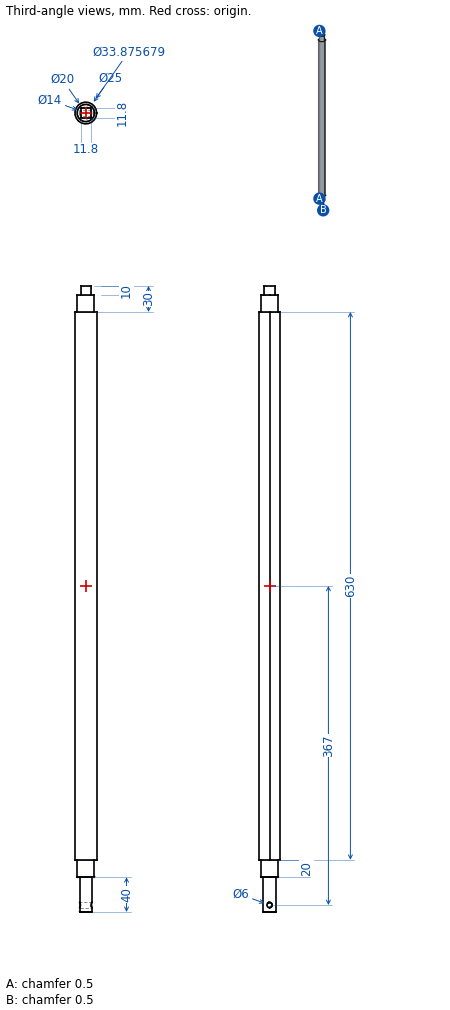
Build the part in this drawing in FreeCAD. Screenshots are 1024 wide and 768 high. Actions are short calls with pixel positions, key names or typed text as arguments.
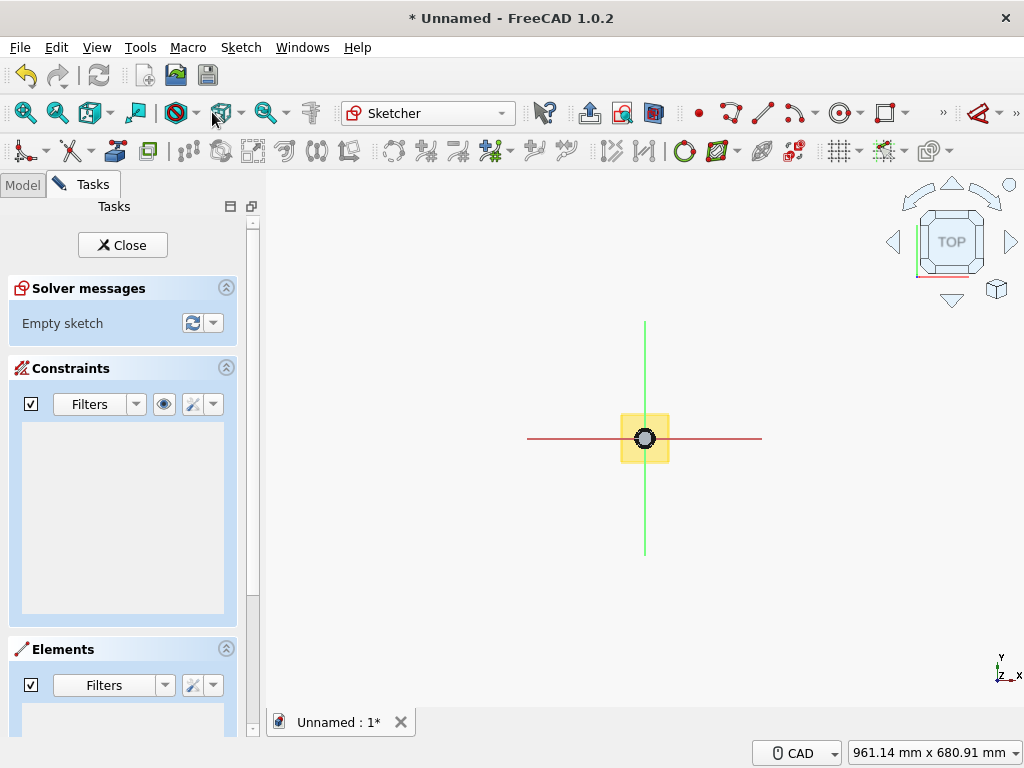
click(654, 114)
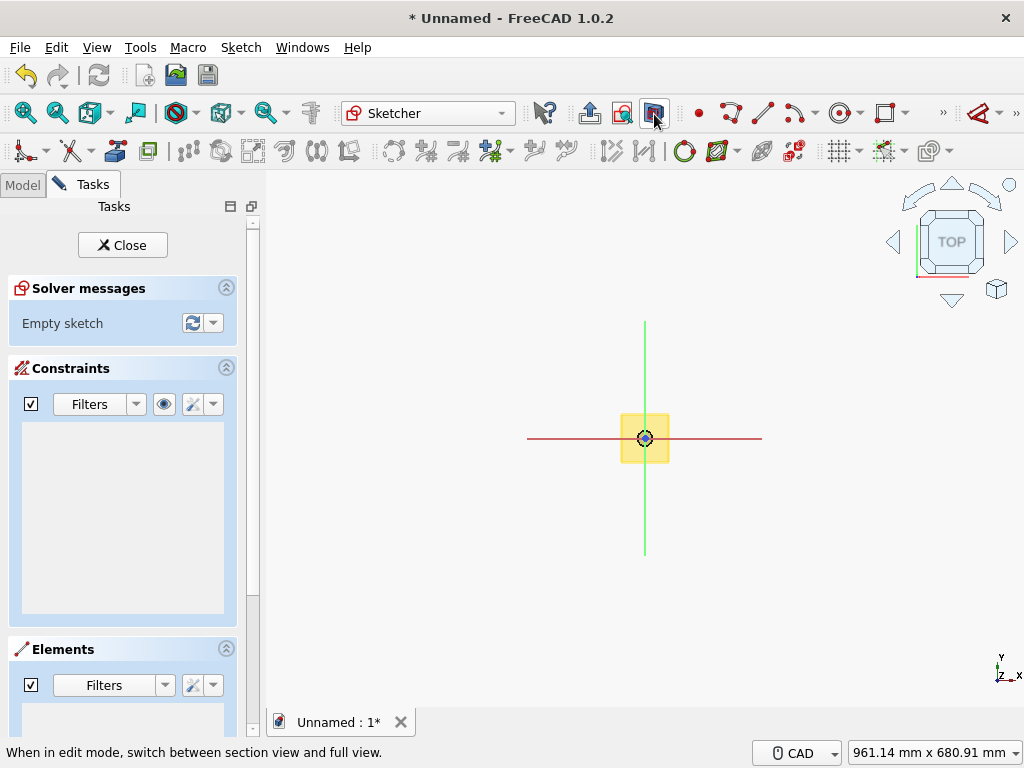
scroll(649, 438, up, 15)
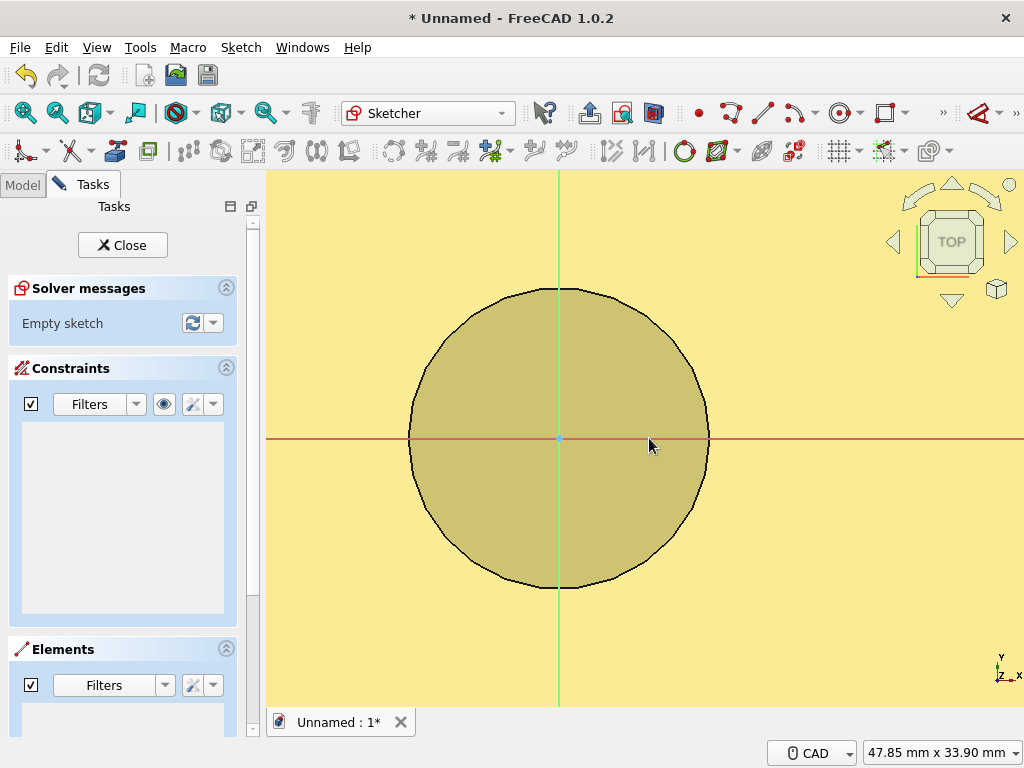
scroll(523, 439, up, 2)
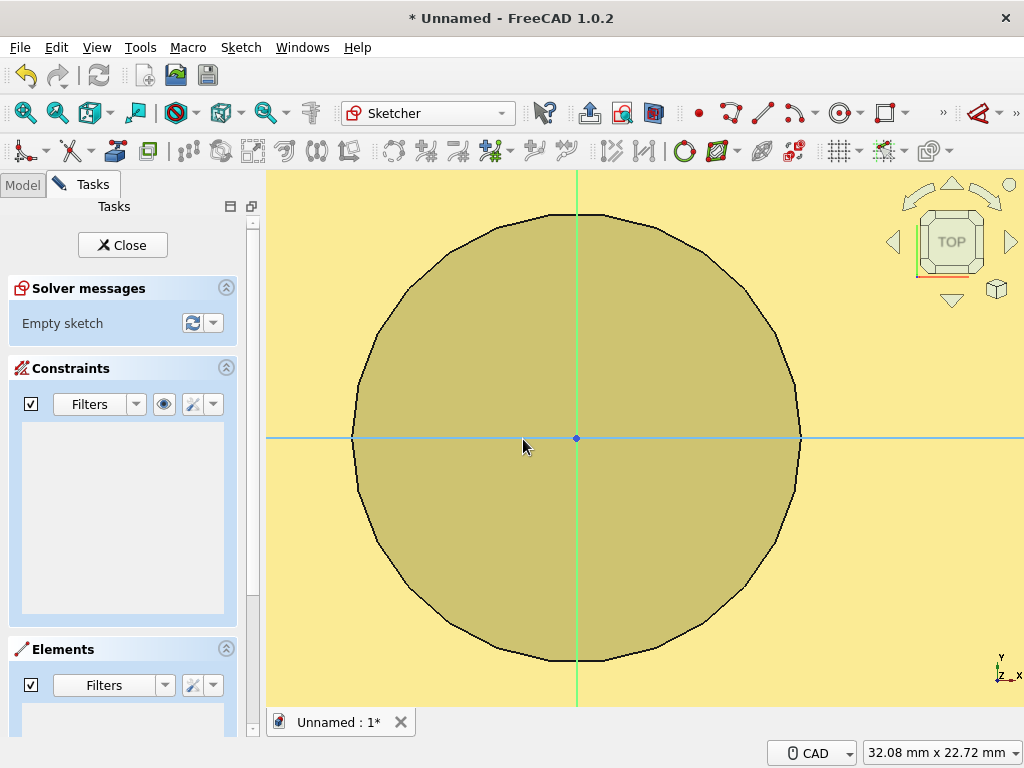
click(840, 114)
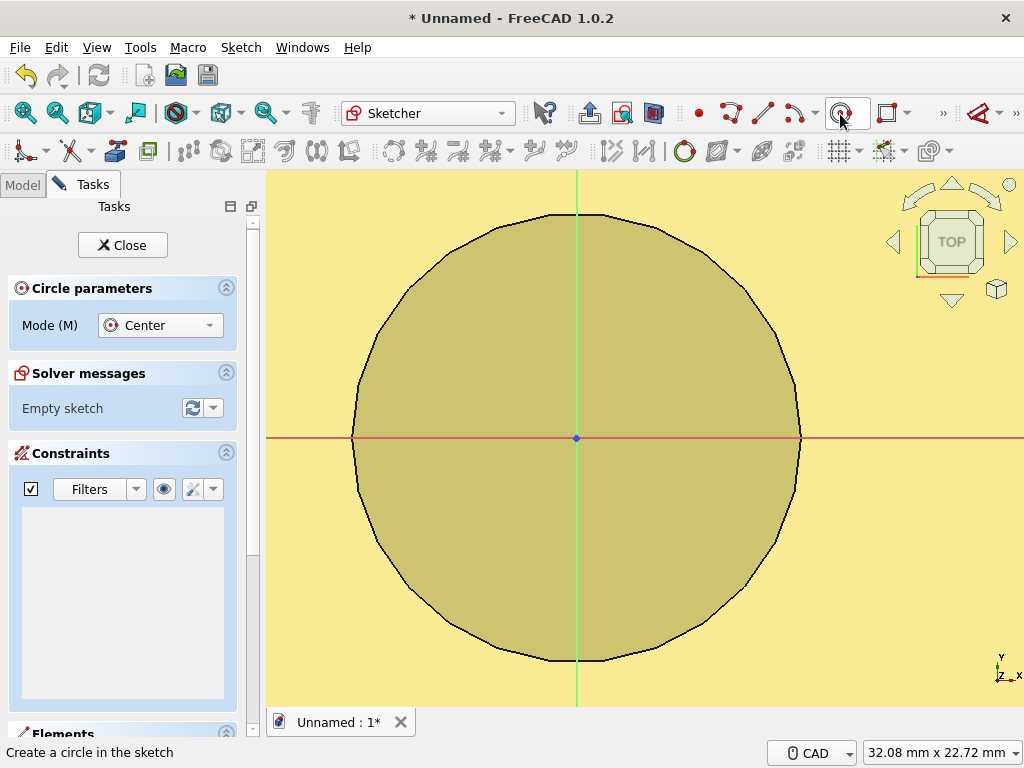
click(577, 438)
move(694, 321)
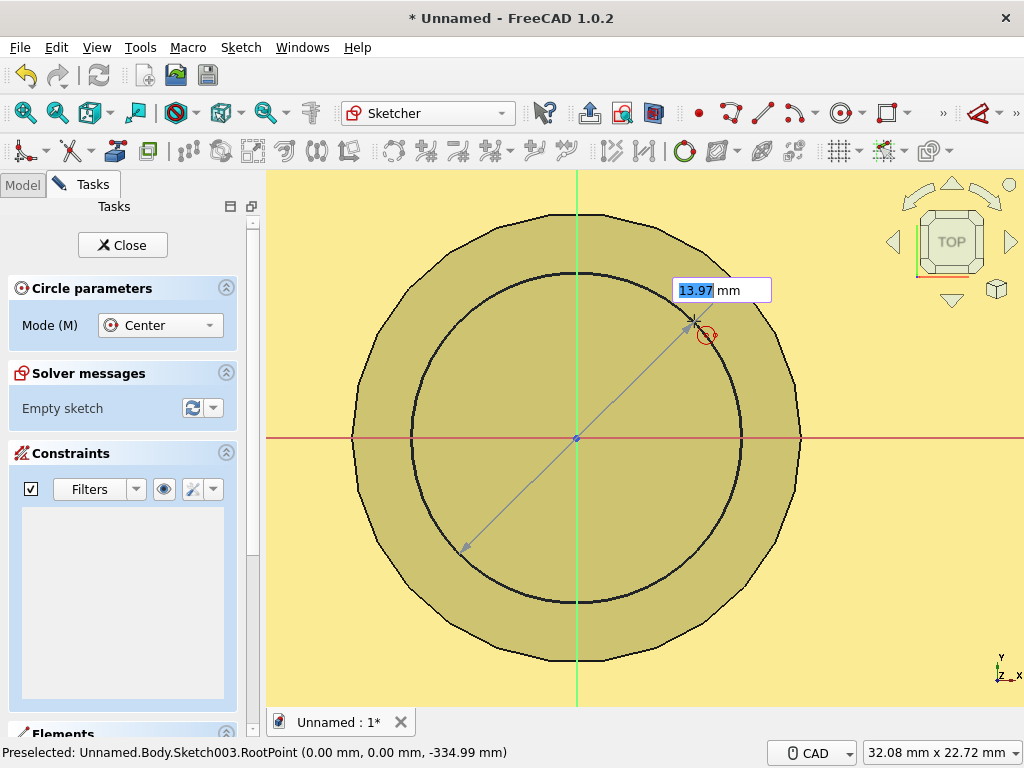
text(14)
key(Return)
key(Escape)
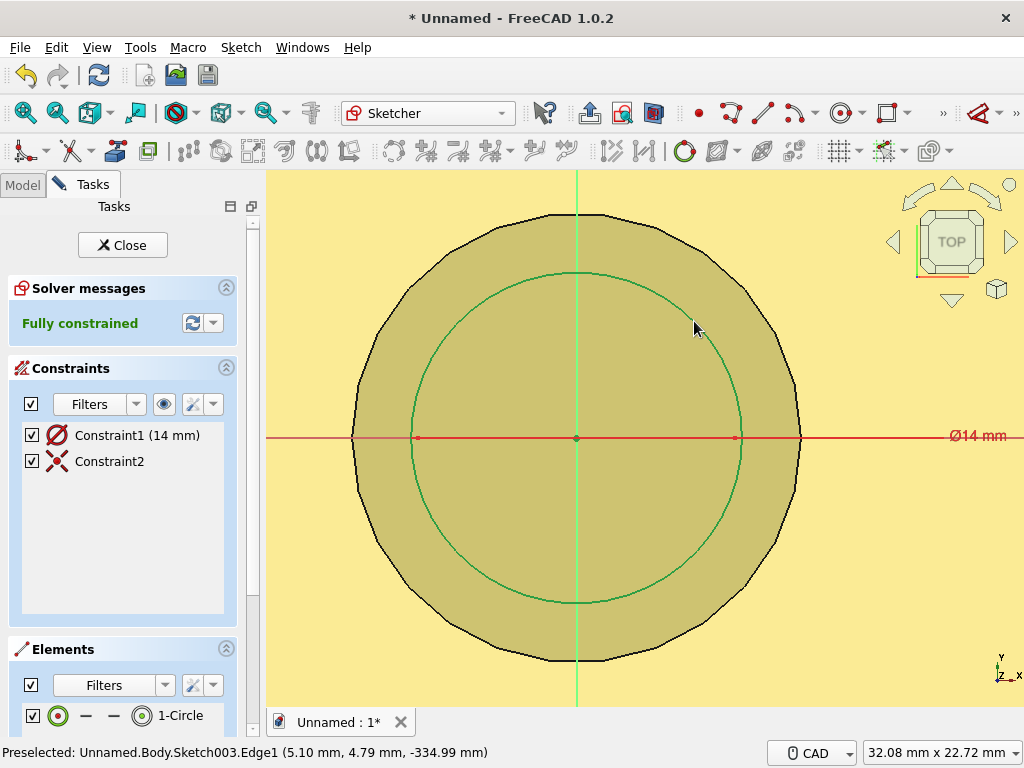
click(123, 245)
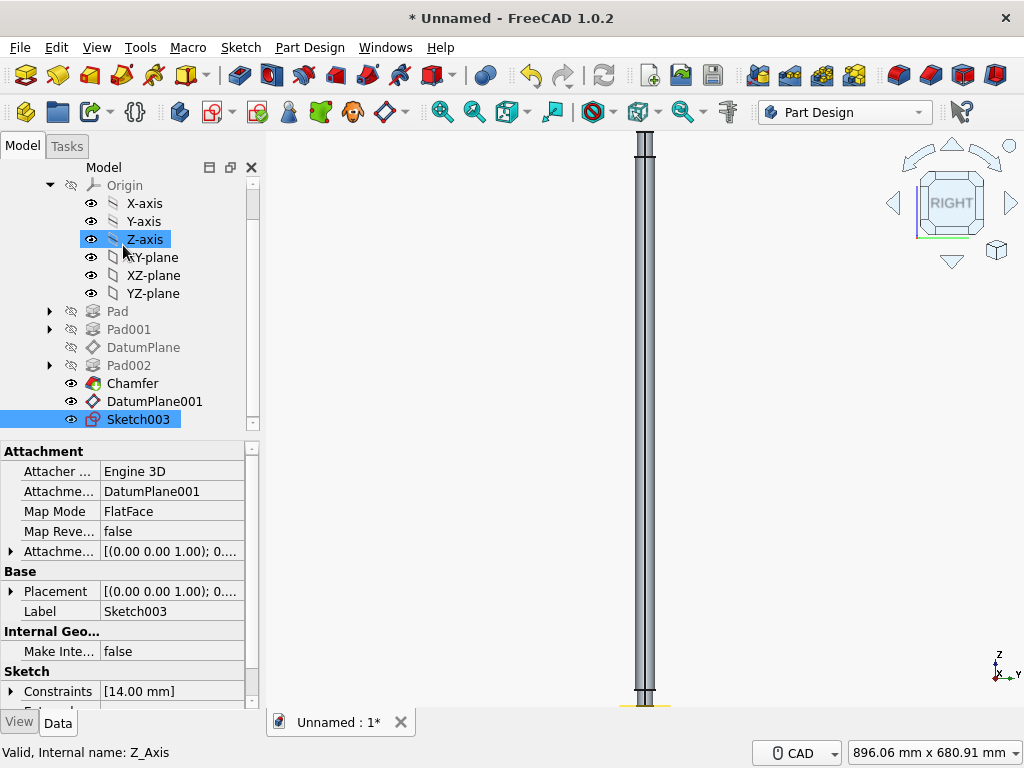
click(26, 76)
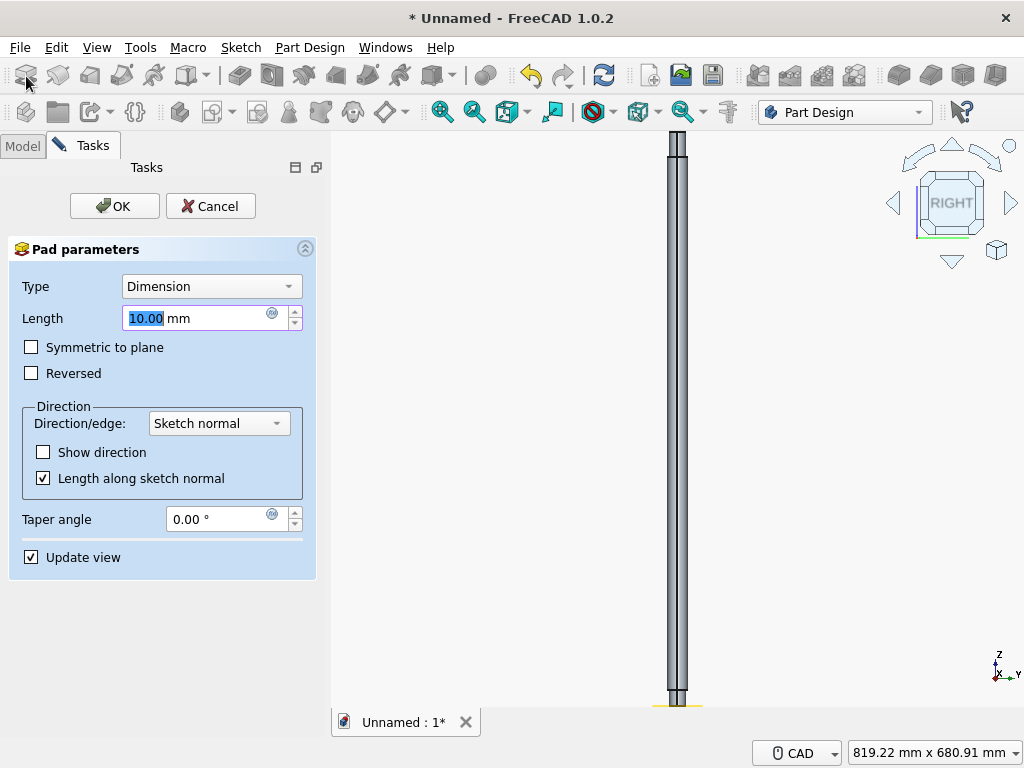
text(40)
key(Tab)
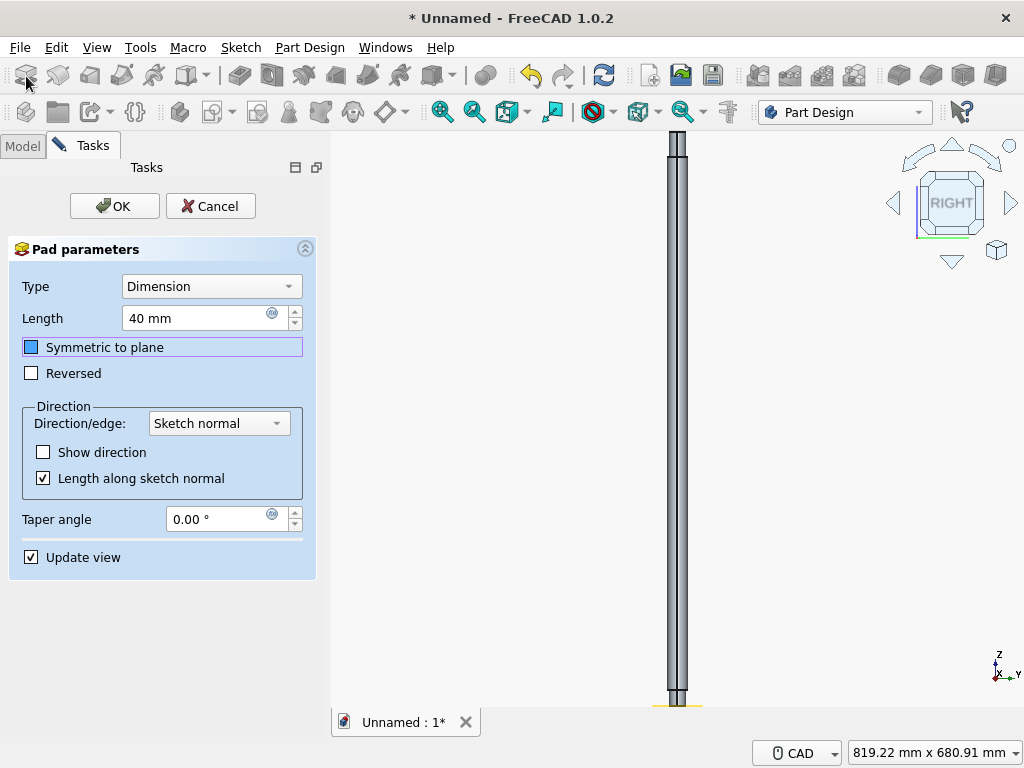
click(30, 373)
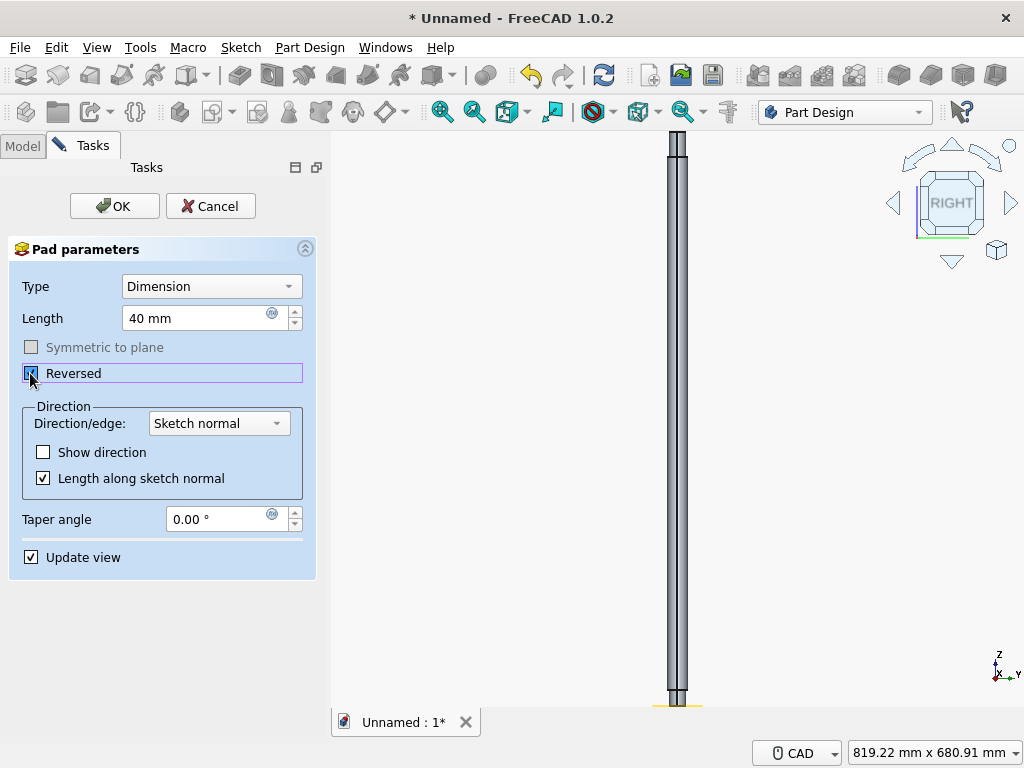
click(115, 206)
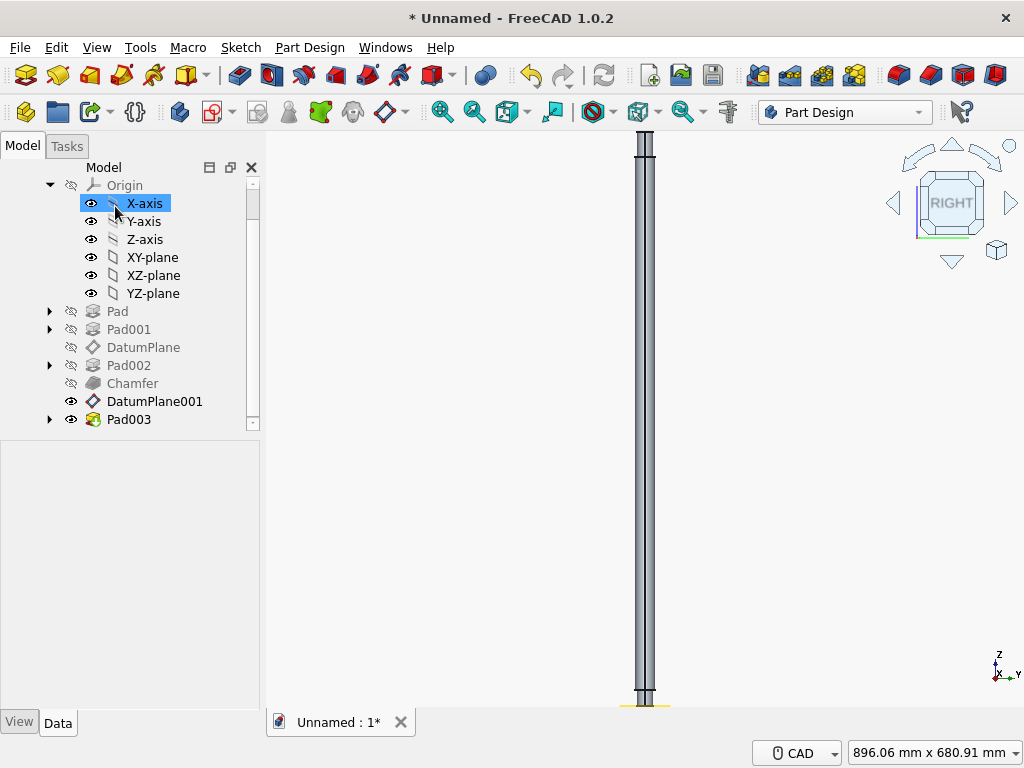
click(116, 401)
key(space)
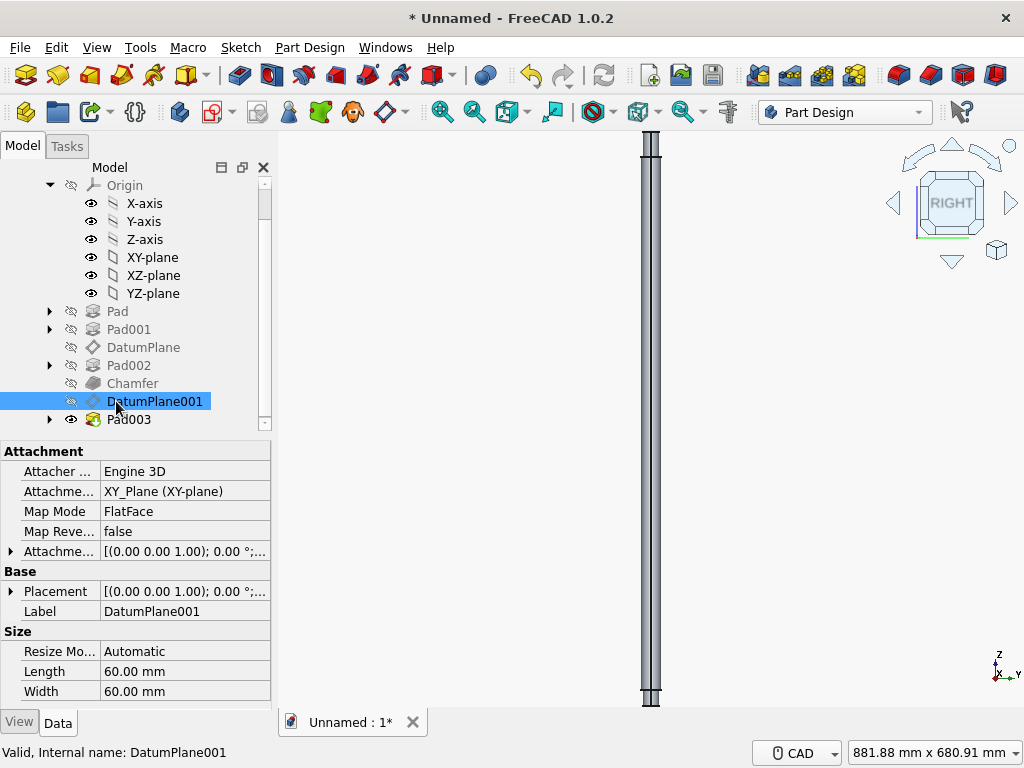
click(444, 112)